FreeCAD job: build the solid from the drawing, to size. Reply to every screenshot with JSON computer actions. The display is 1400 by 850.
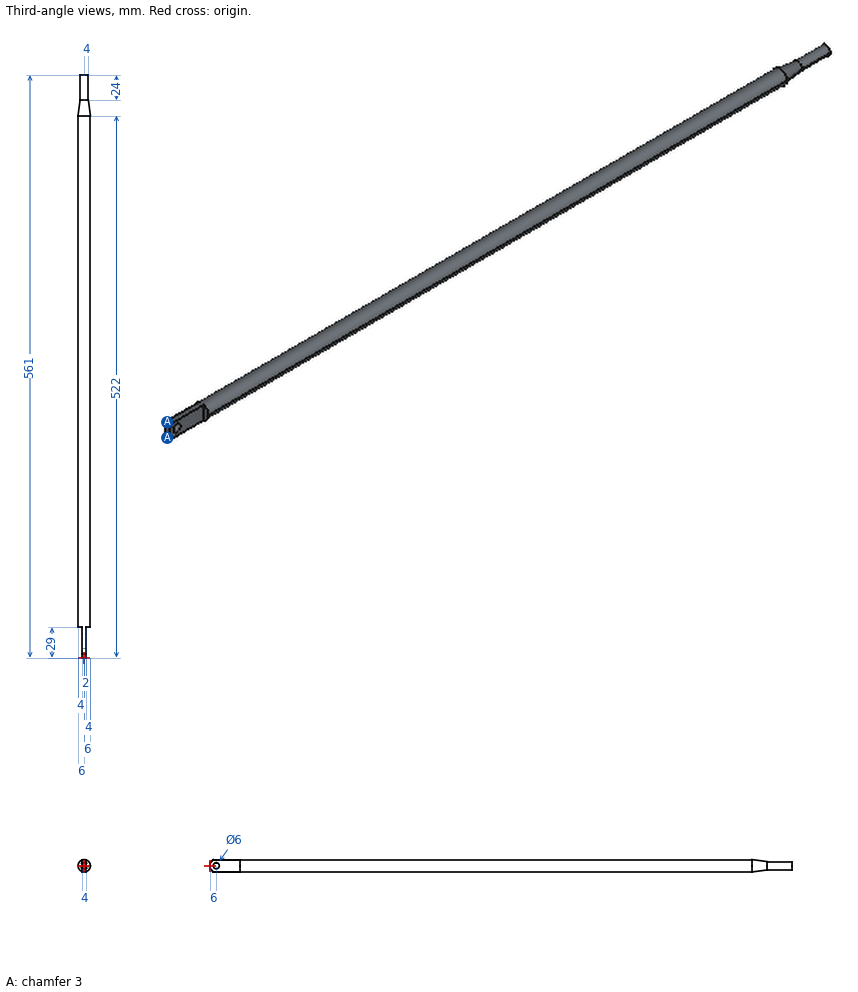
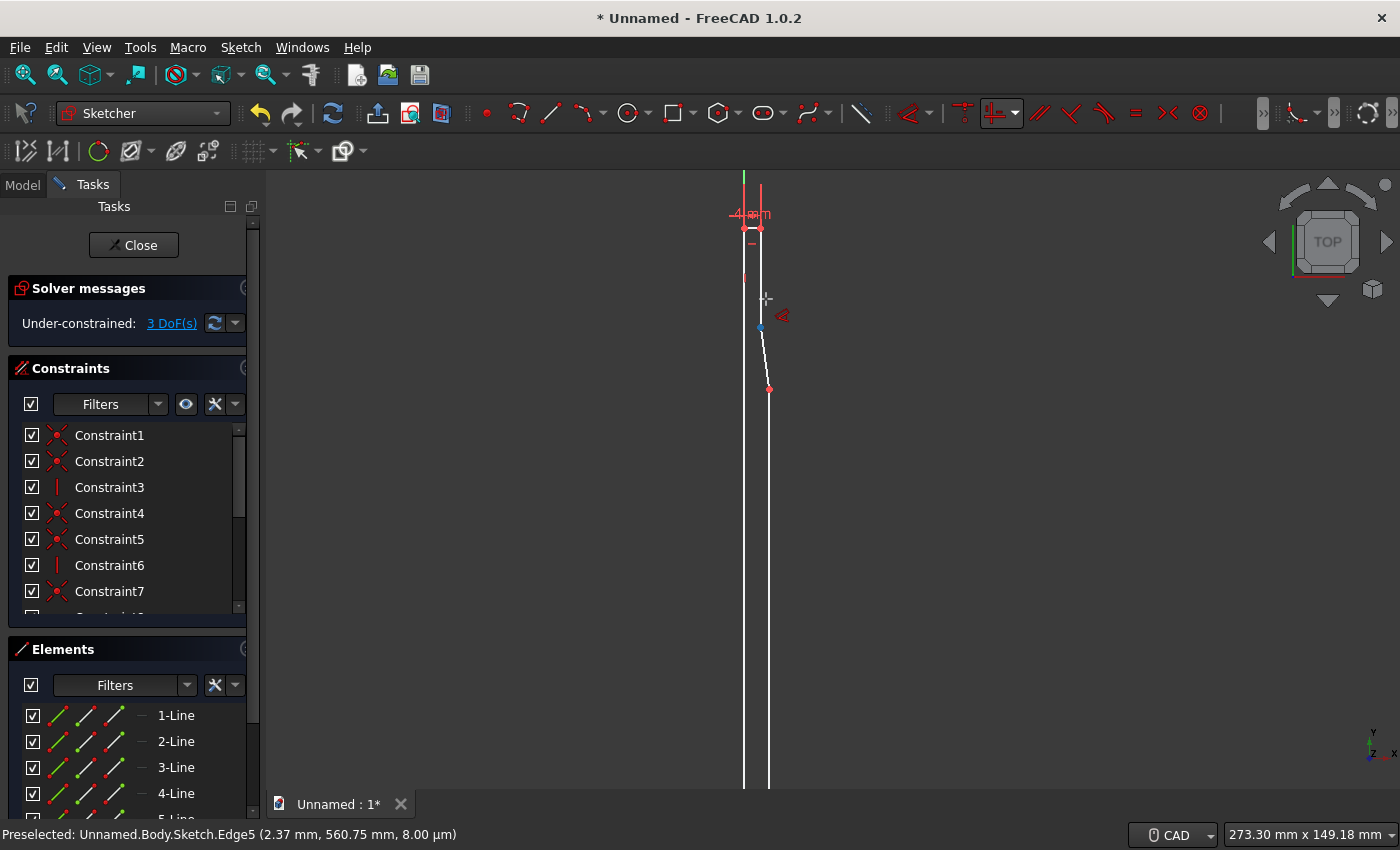
{"action": "left_click", "coordinate": [761, 298]}
{"action": "left_click", "coordinate": [795, 278]}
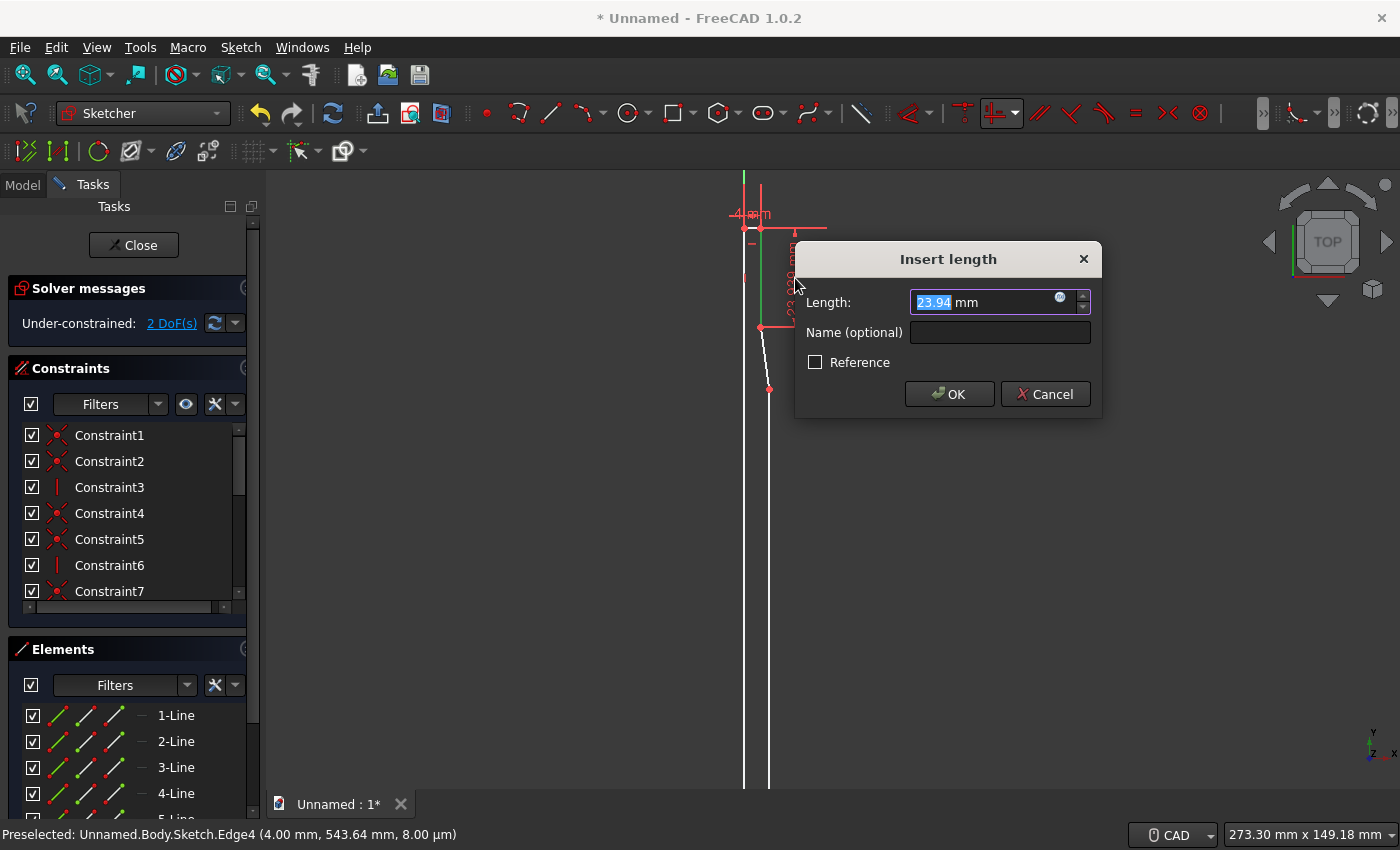
{"action": "type", "text": "24"}
{"action": "key", "text": "Return"}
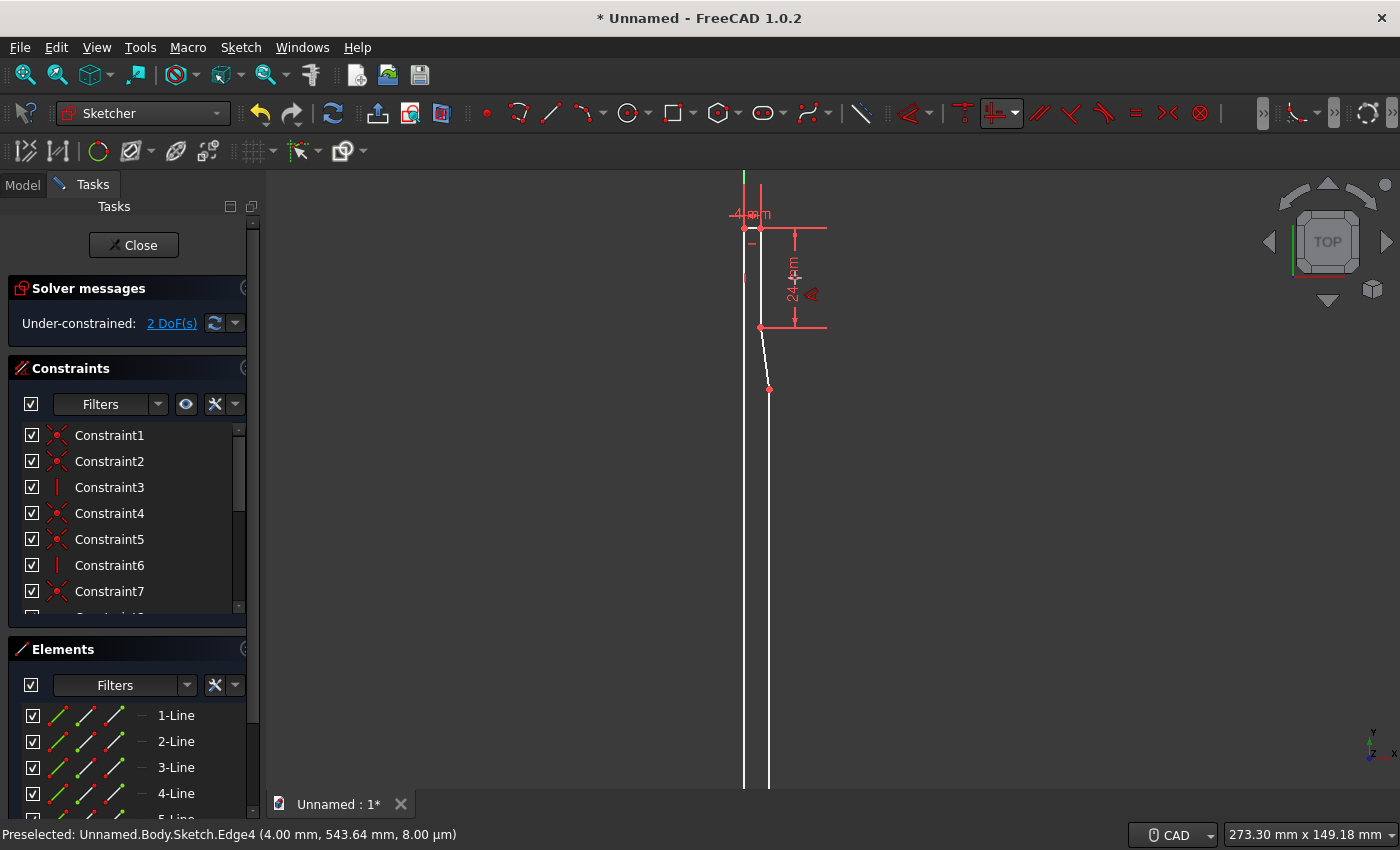
{"action": "scroll", "coordinate": [766, 299], "scroll_direction": "down", "scroll_amount": 9}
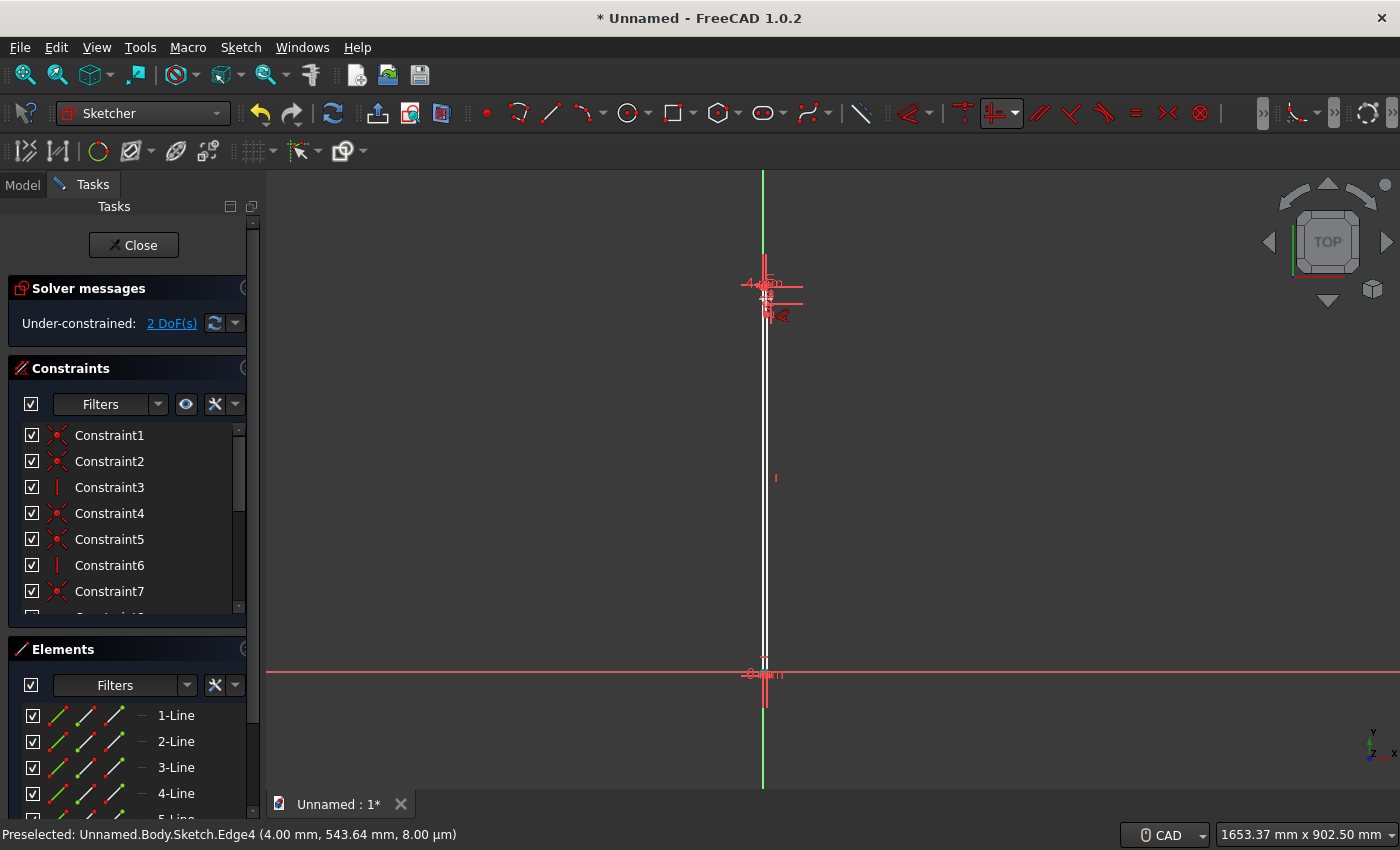
{"action": "scroll", "coordinate": [767, 565], "scroll_direction": "up", "scroll_amount": 7}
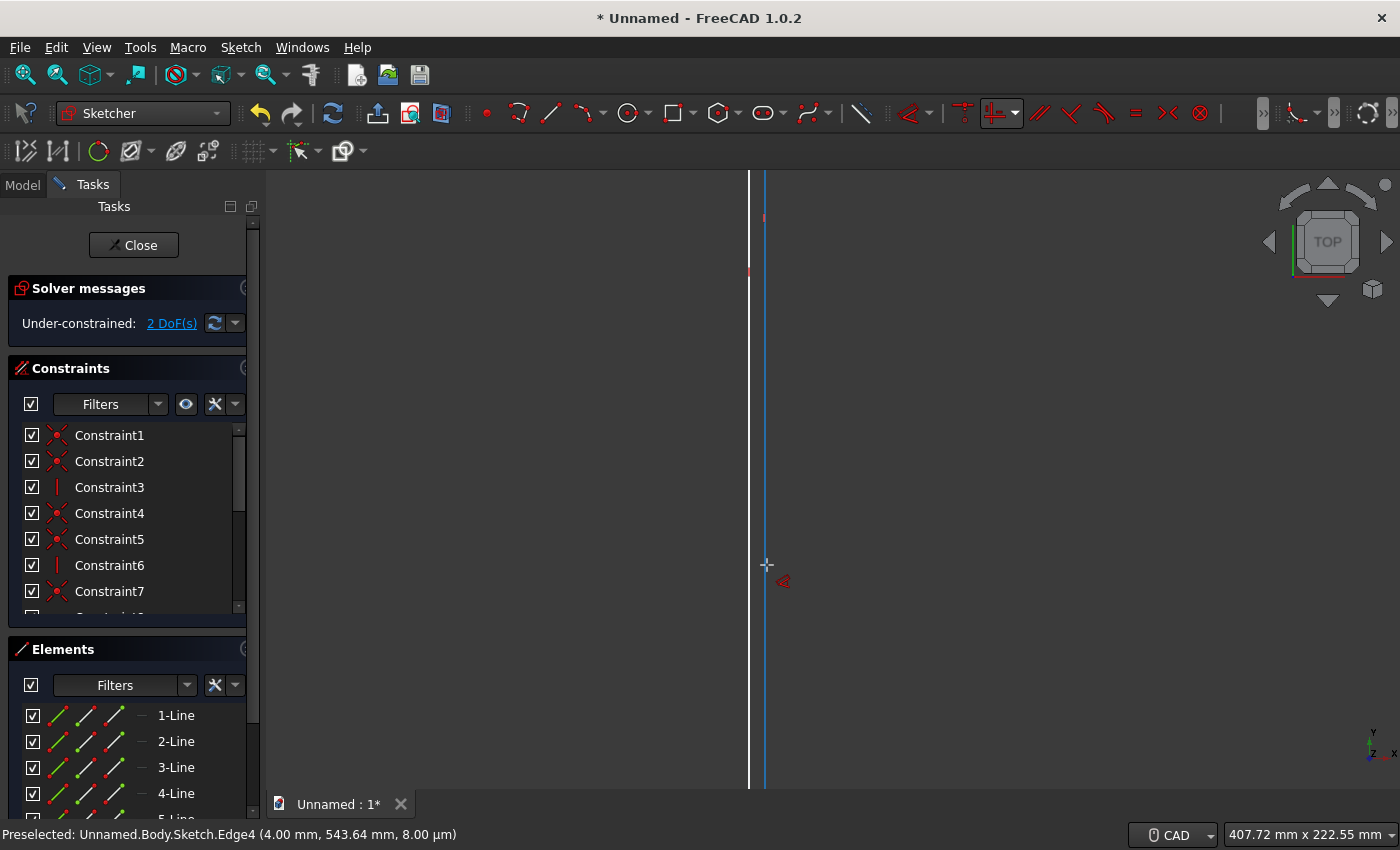
{"action": "left_click", "coordinate": [765, 562]}
{"action": "left_click", "coordinate": [799, 480]}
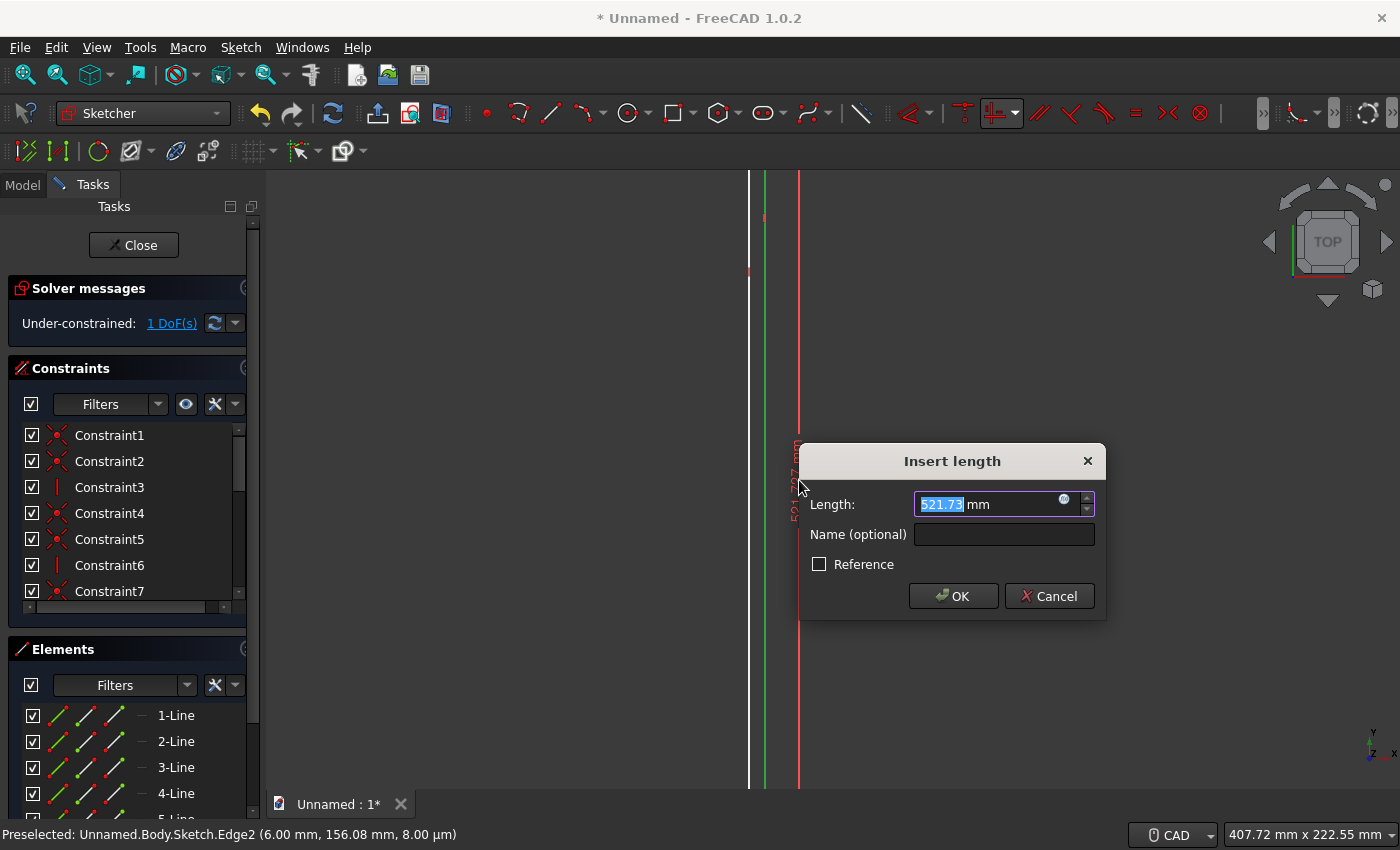
{"action": "type", "text": "522"}
{"action": "key", "text": "Return"}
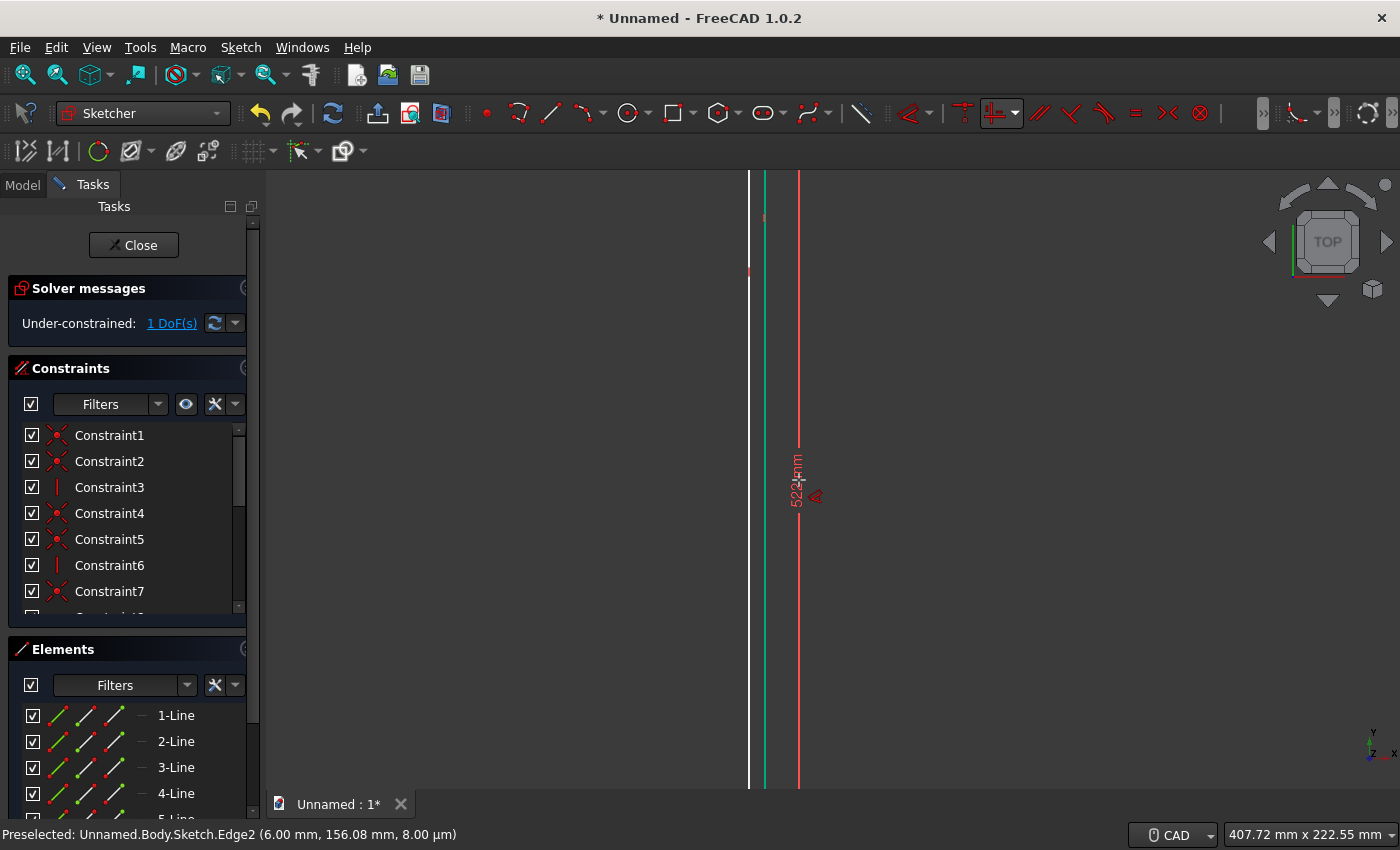
{"action": "left_click", "coordinate": [749, 529]}
{"action": "left_click", "coordinate": [715, 480]}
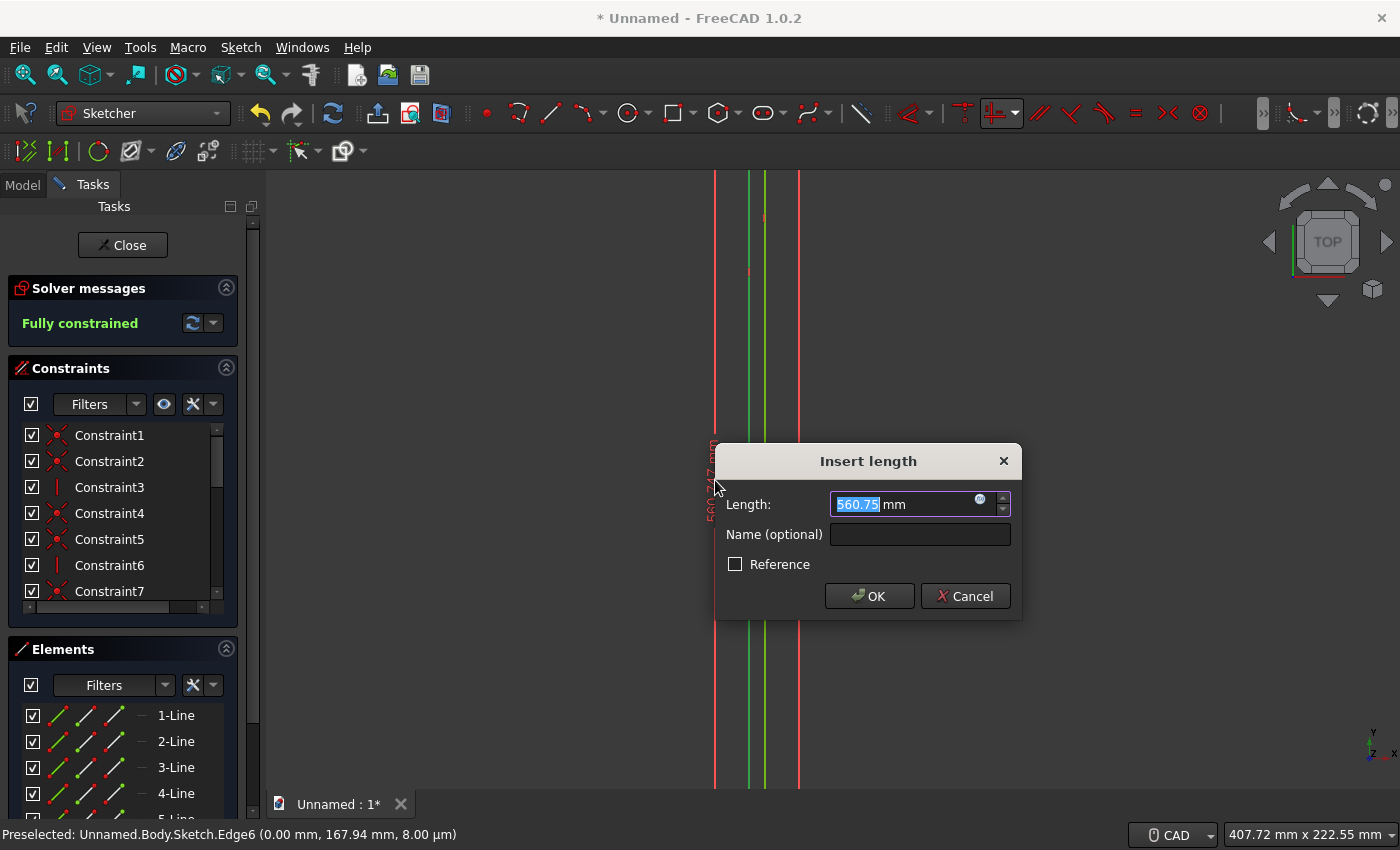
{"action": "type", "text": "561"}
{"action": "key", "text": "Return"}
{"action": "key", "text": "Escape"}